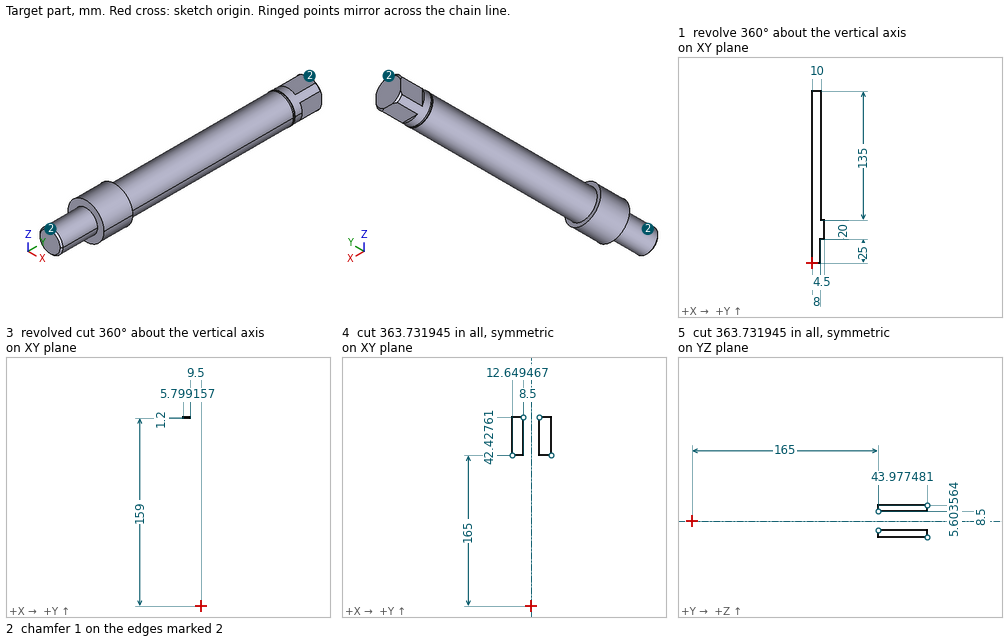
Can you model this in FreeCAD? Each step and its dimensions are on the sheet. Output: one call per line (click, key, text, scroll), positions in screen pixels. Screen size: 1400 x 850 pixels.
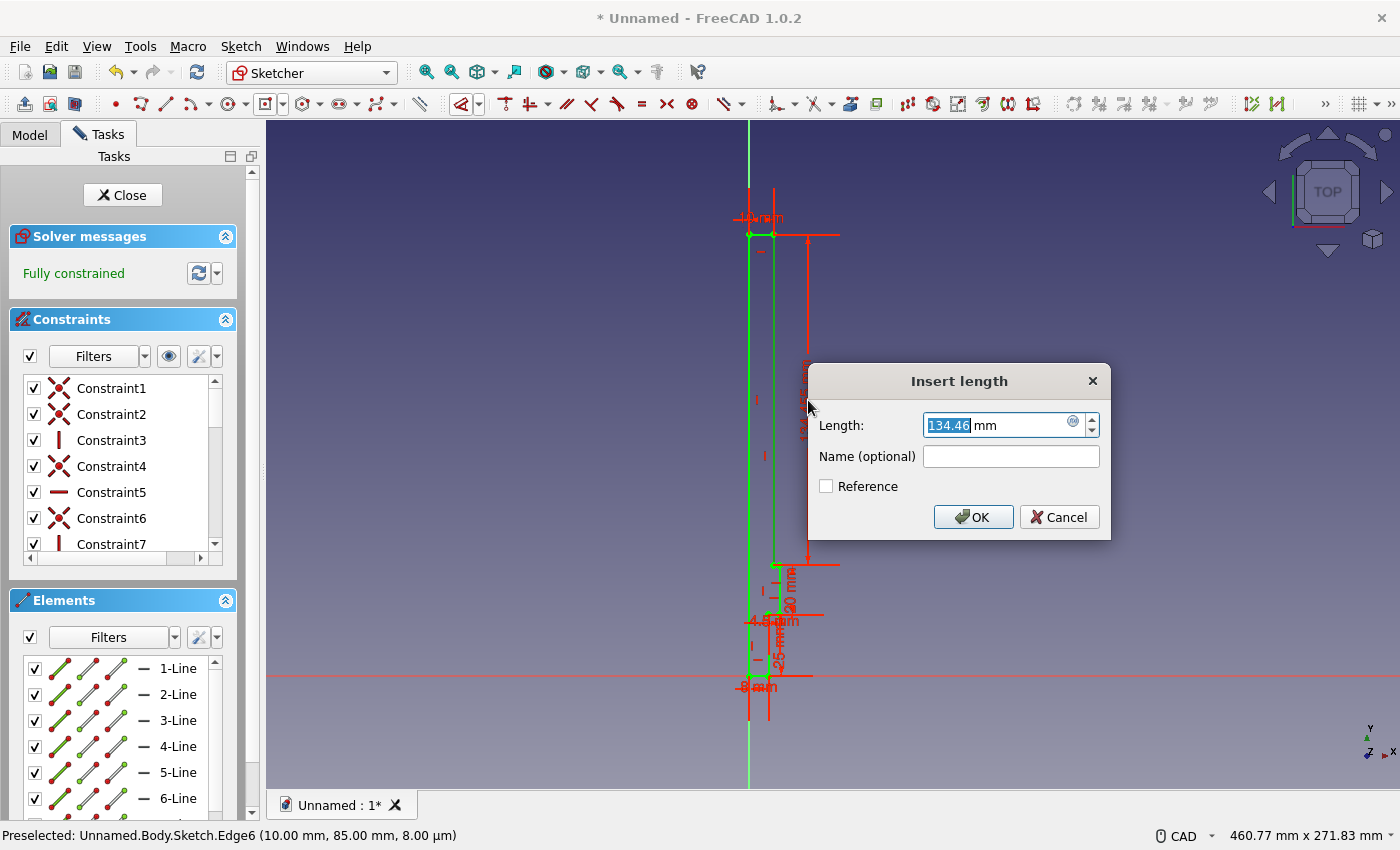
text(135)
key(Return)
key(Escape)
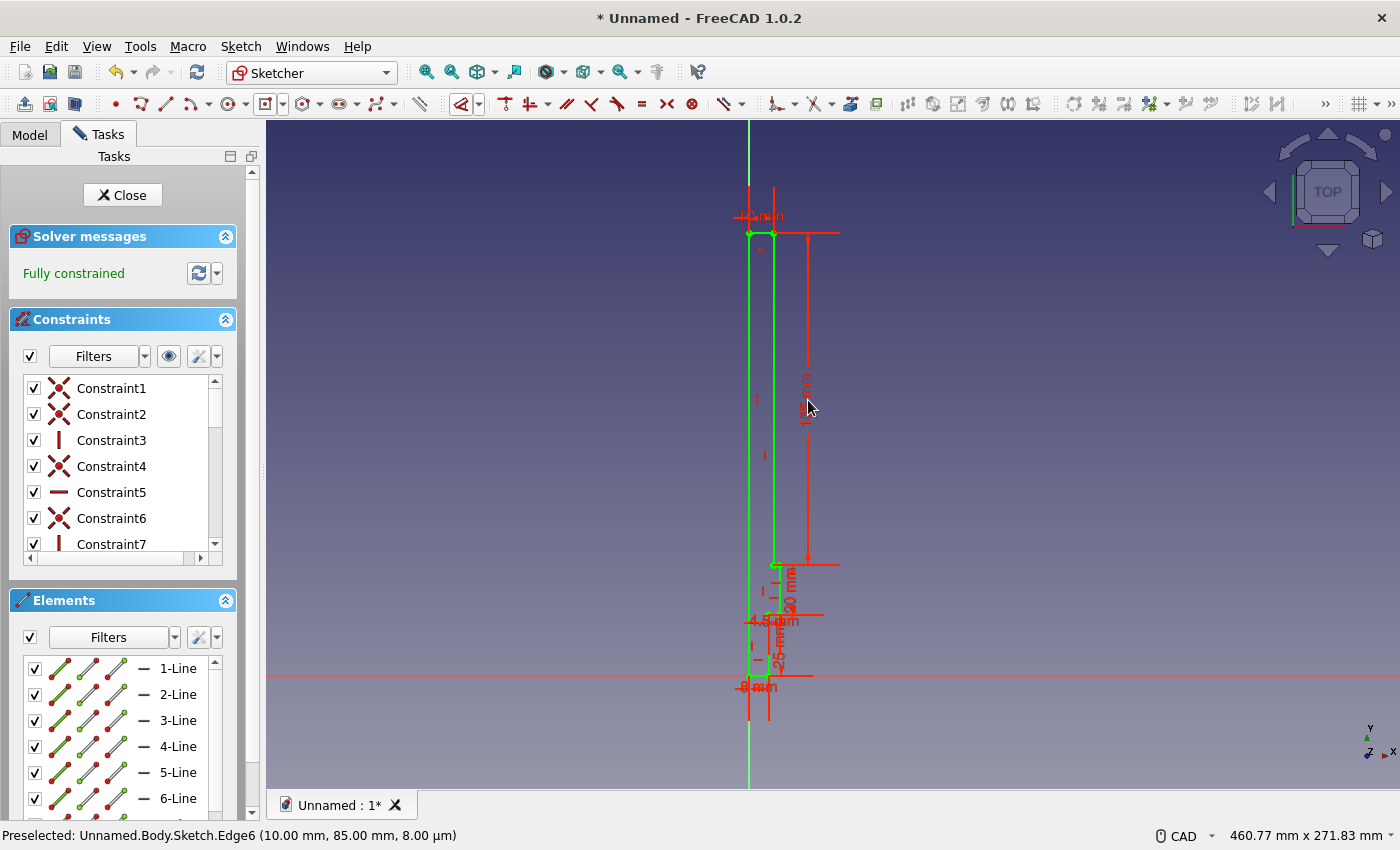
click(123, 195)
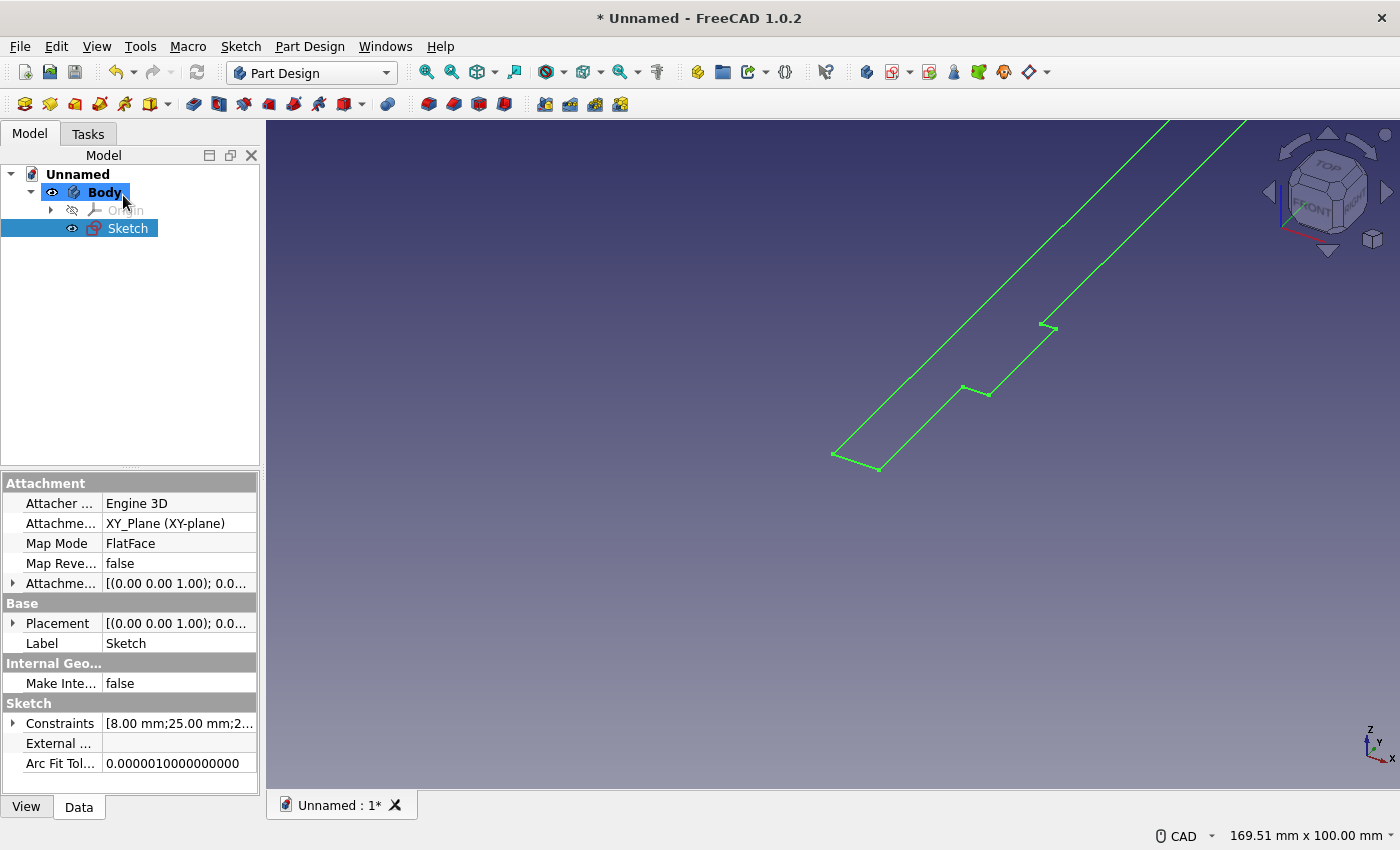
click(50, 104)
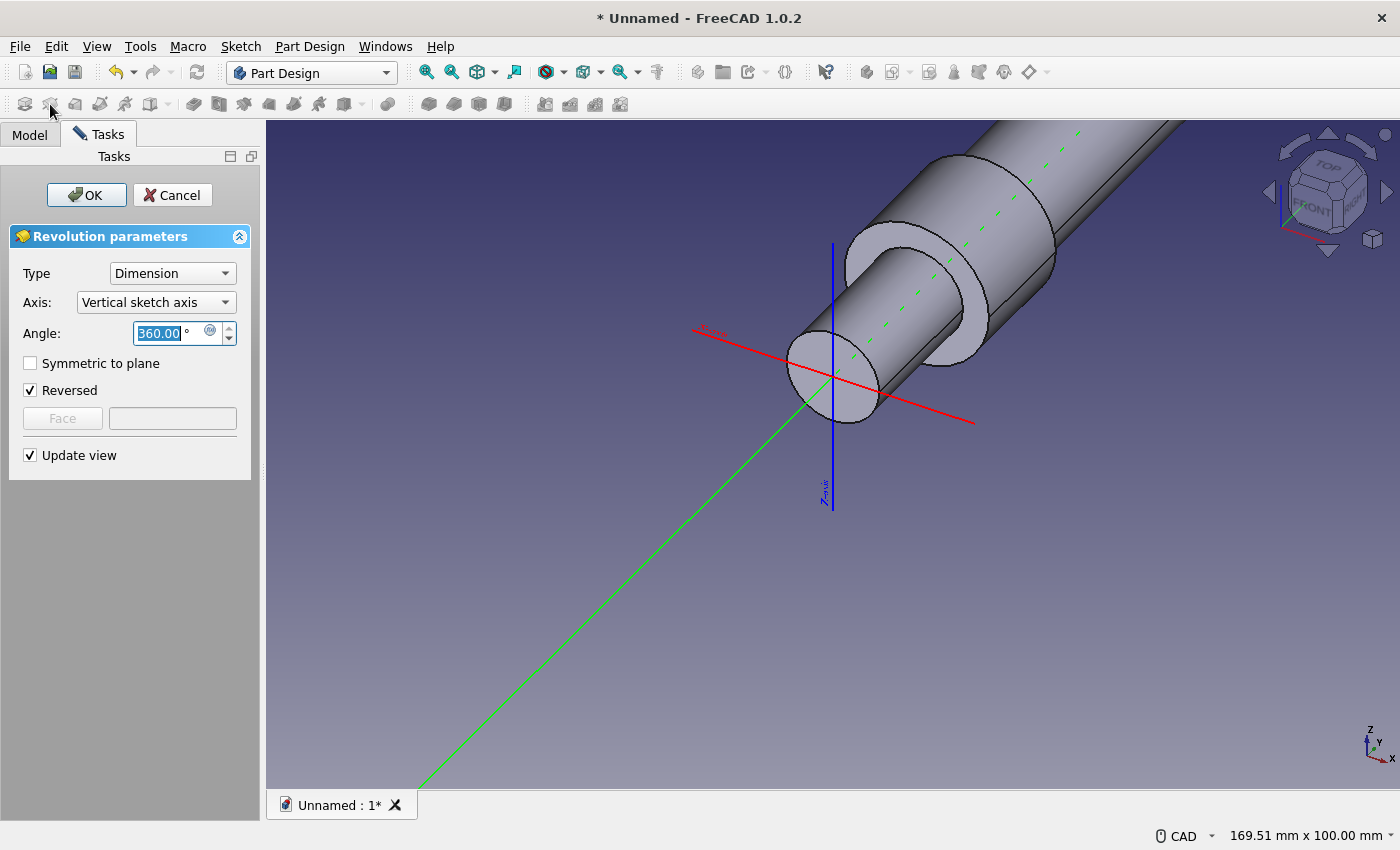
click(87, 195)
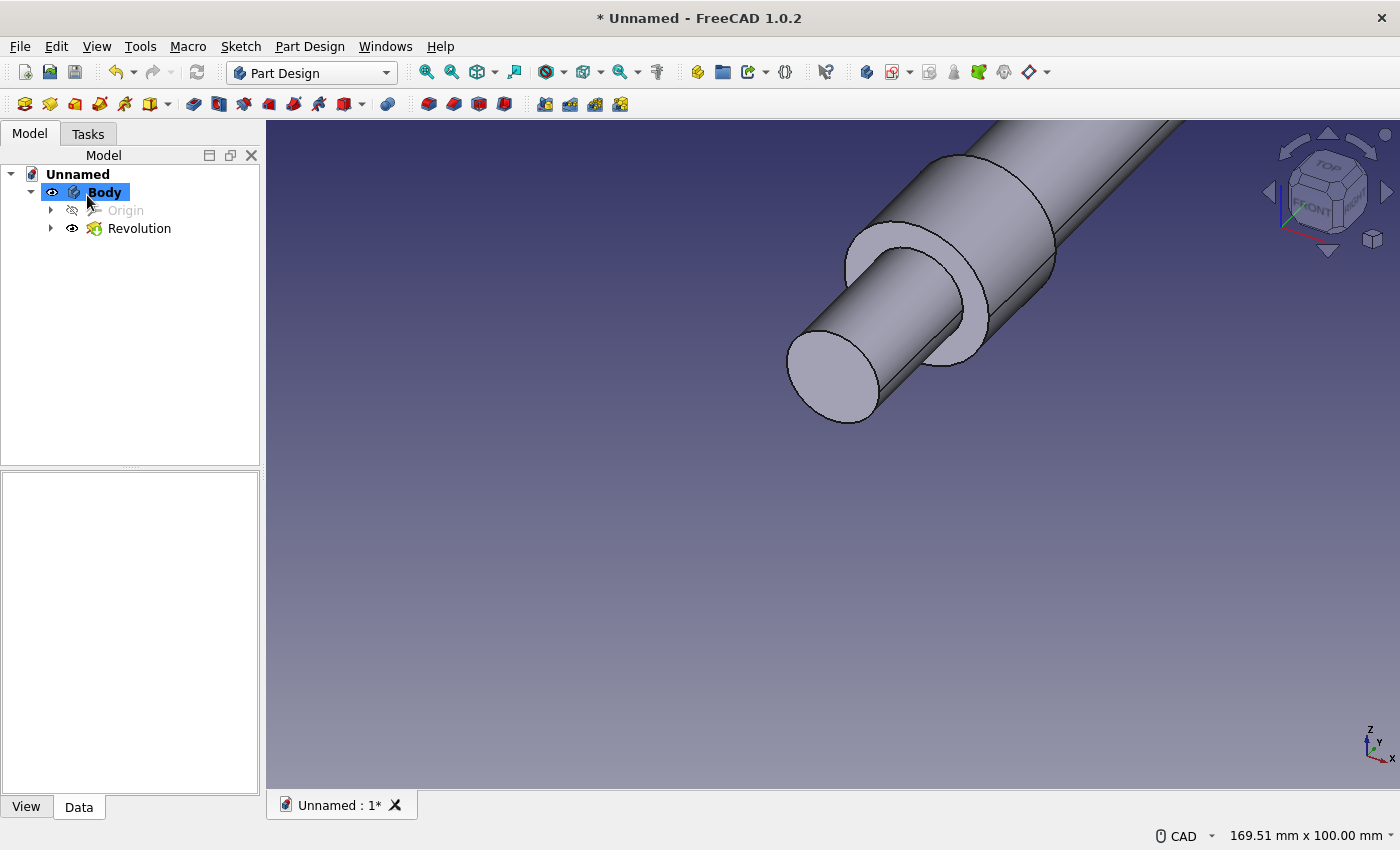
key(v)
key(f)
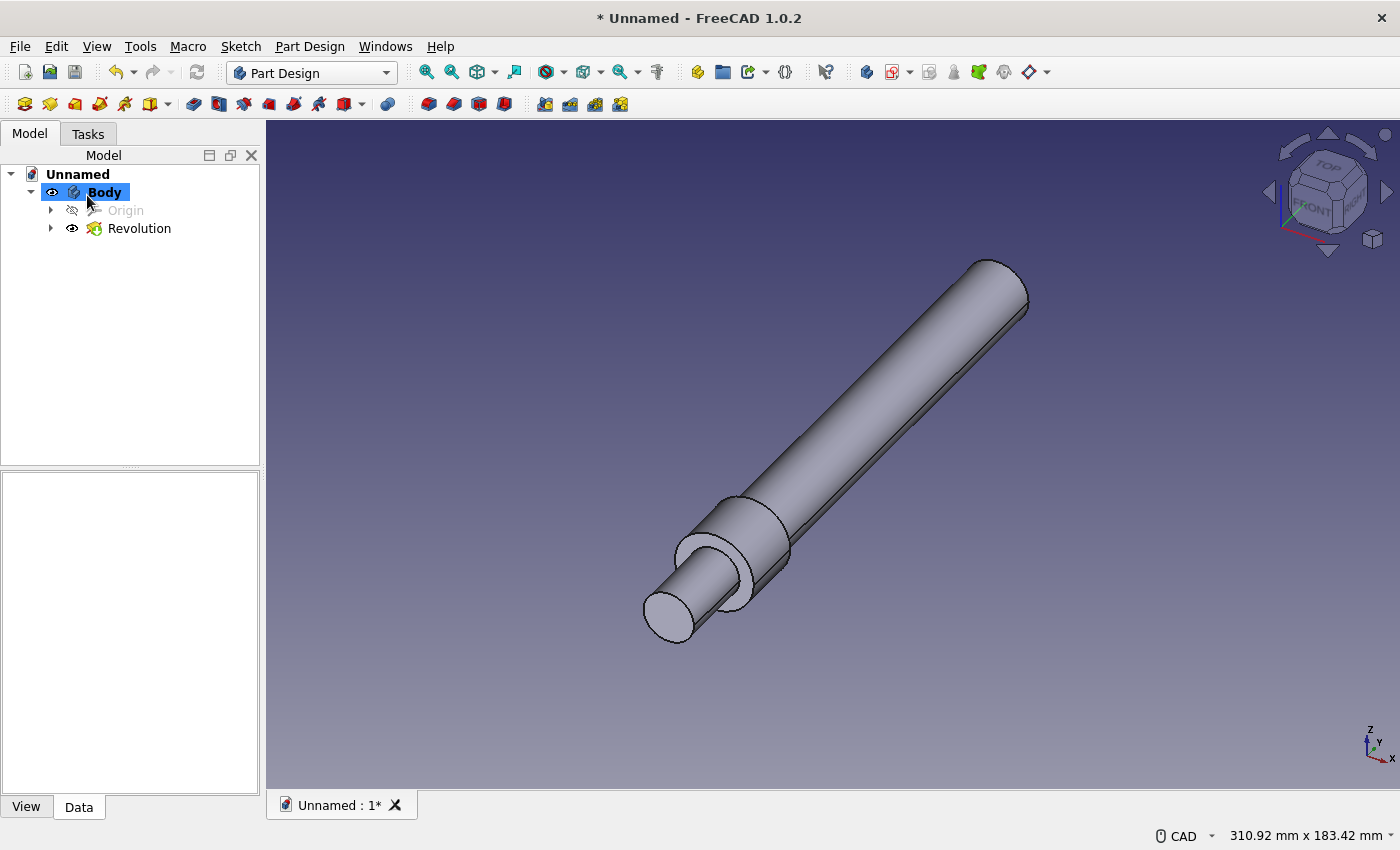
click(648, 596)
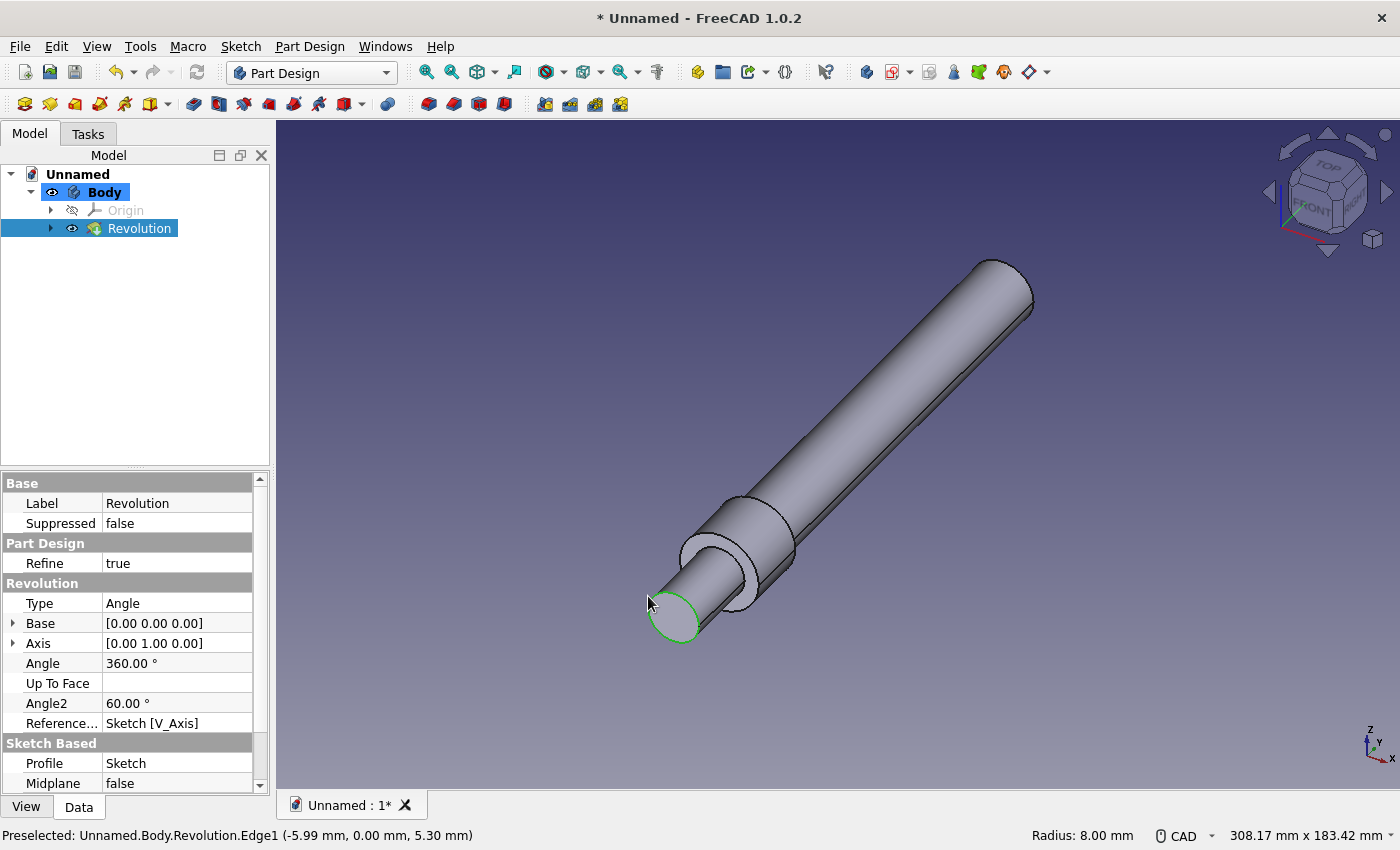
key(0)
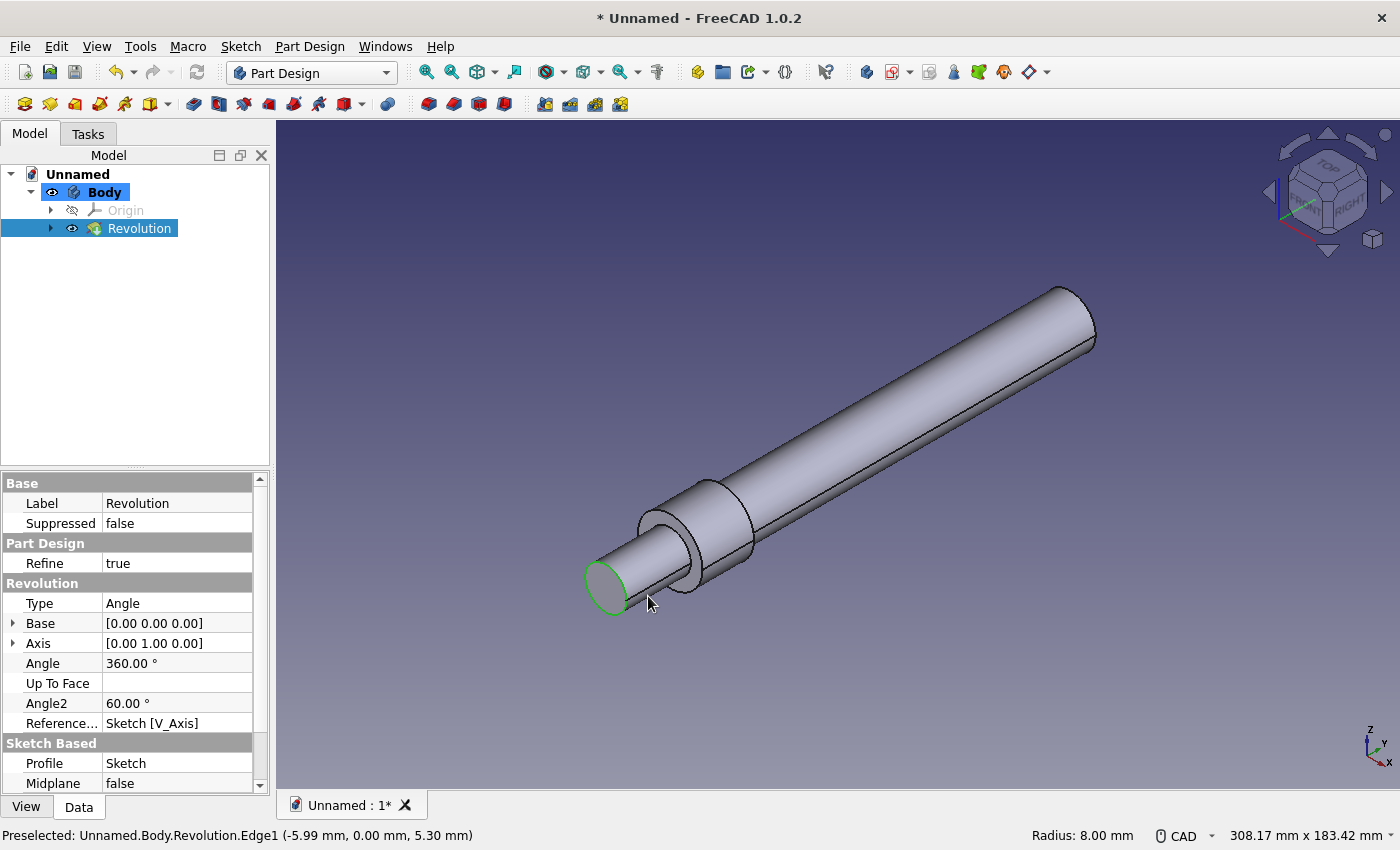
key(2)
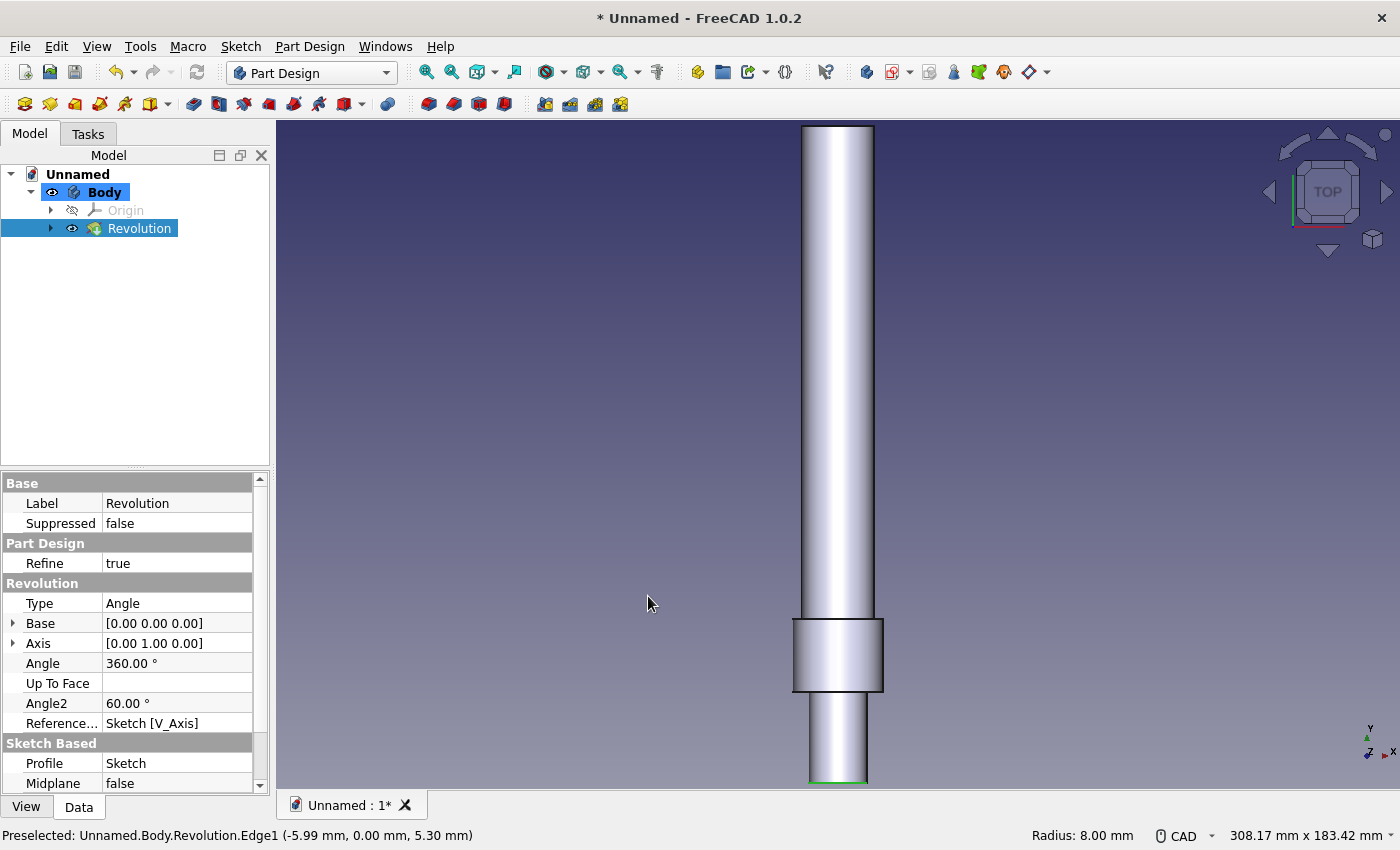
key(1)